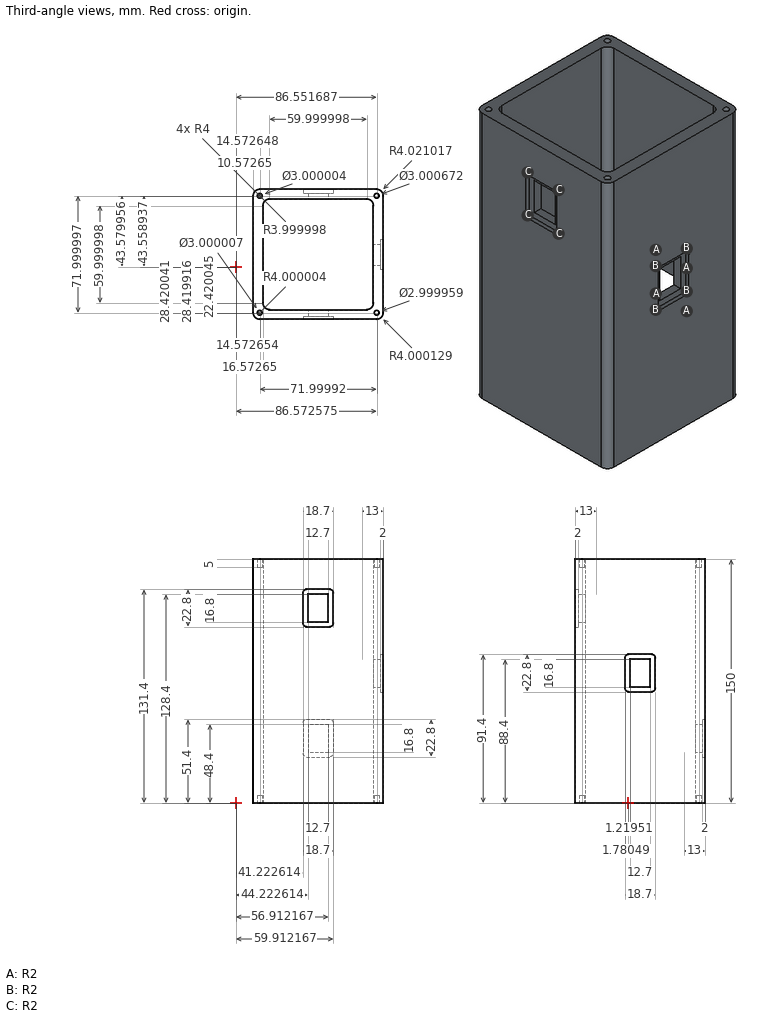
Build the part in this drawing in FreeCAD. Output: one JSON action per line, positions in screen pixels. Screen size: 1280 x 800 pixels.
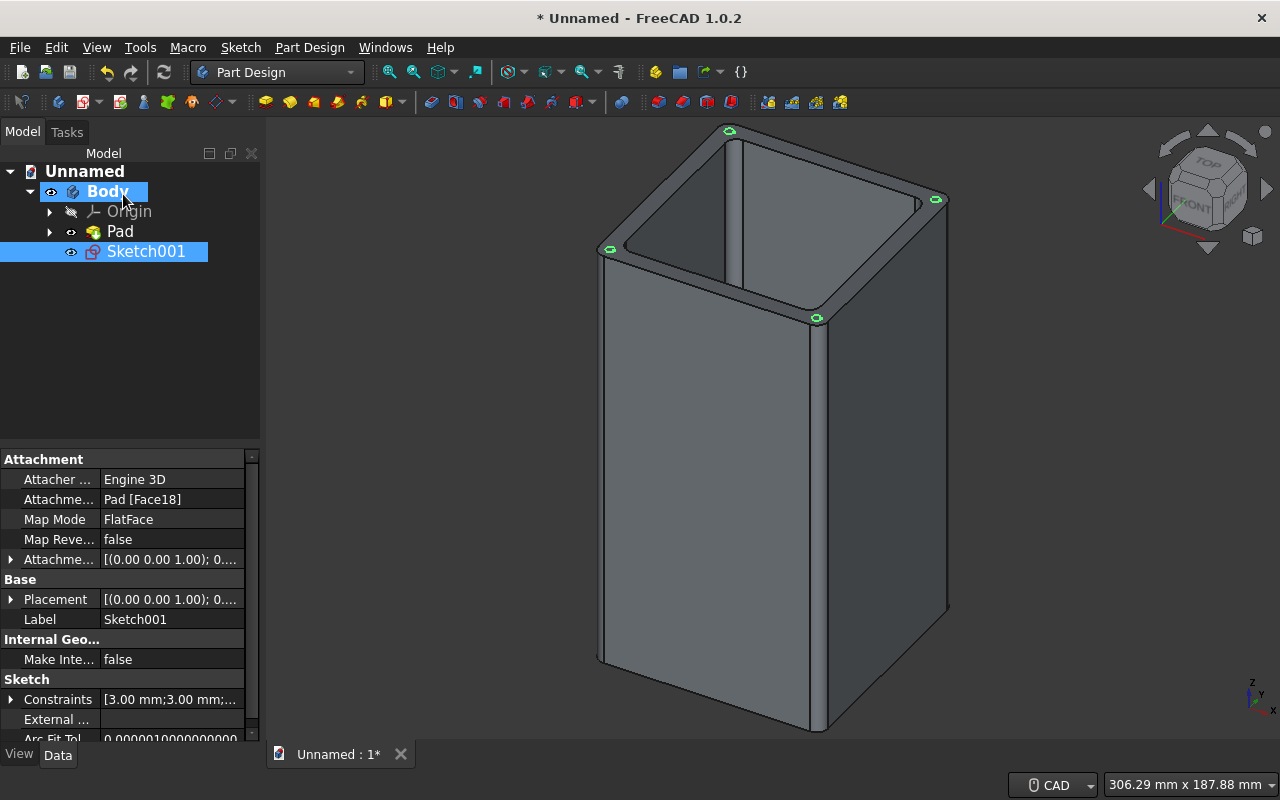
{"action": "left_click", "coordinate": [432, 102]}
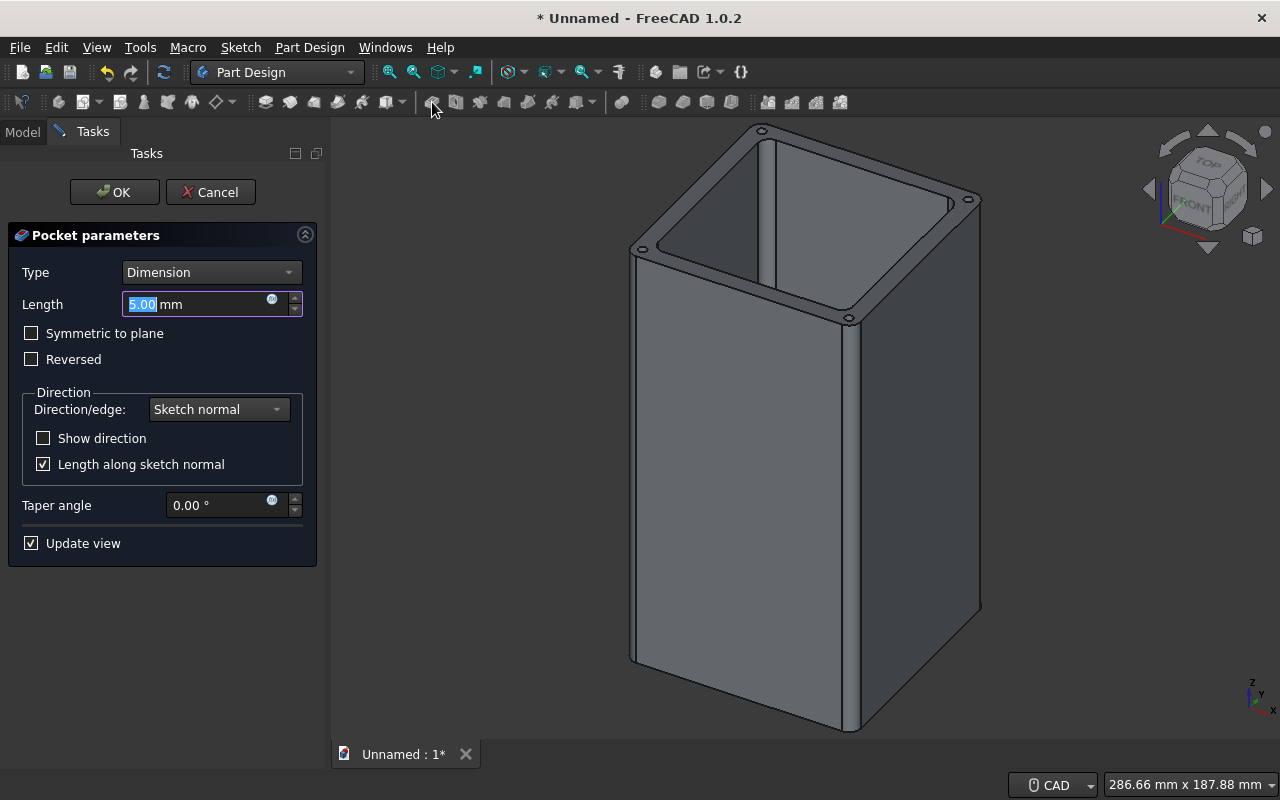
{"action": "type", "text": "5"}
{"action": "key", "text": "Tab"}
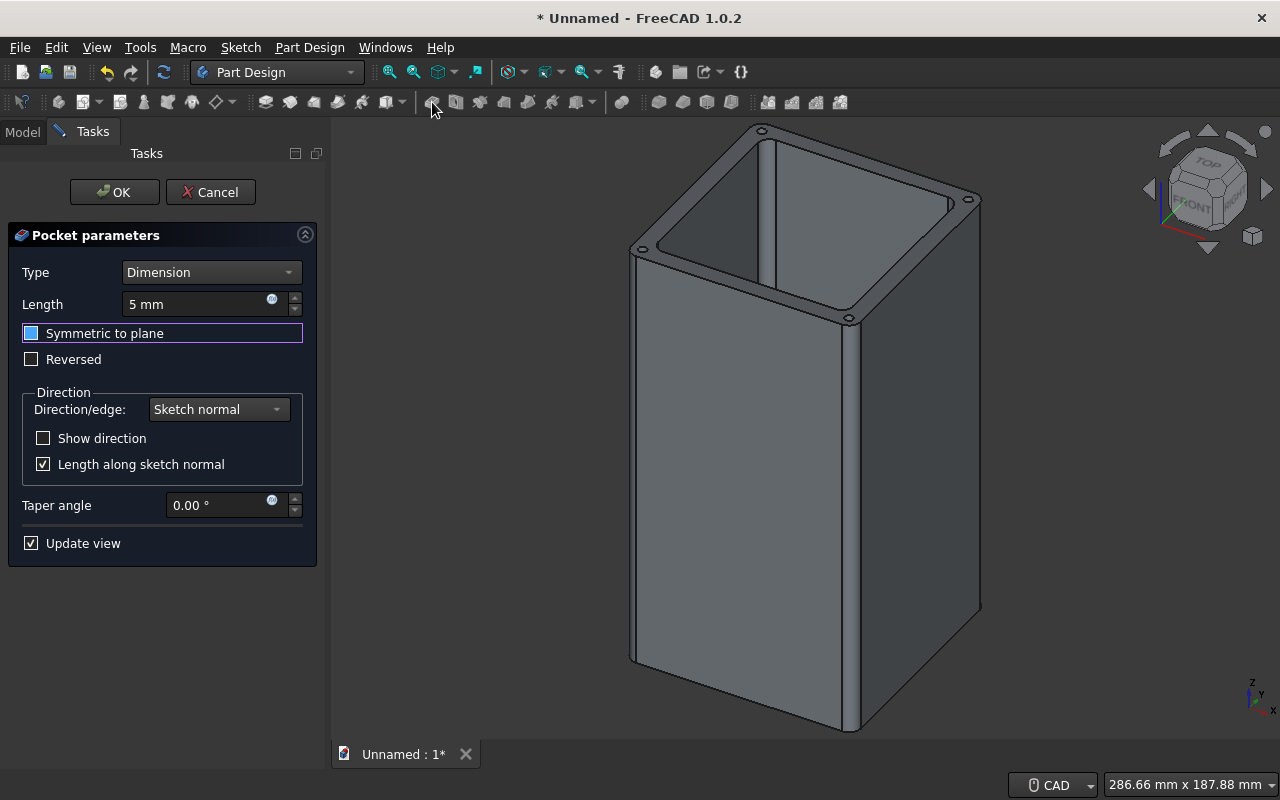
{"action": "left_click", "coordinate": [115, 192]}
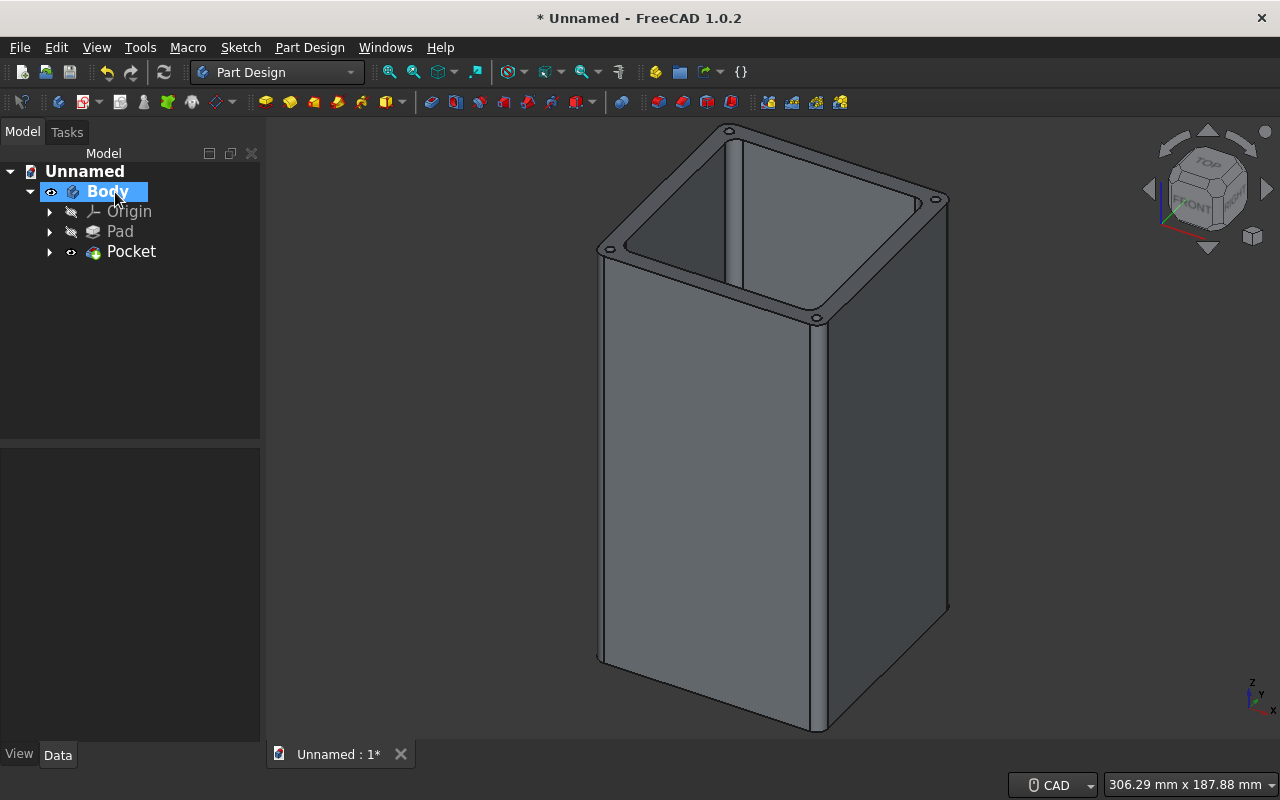
{"action": "left_click", "coordinate": [50, 212]}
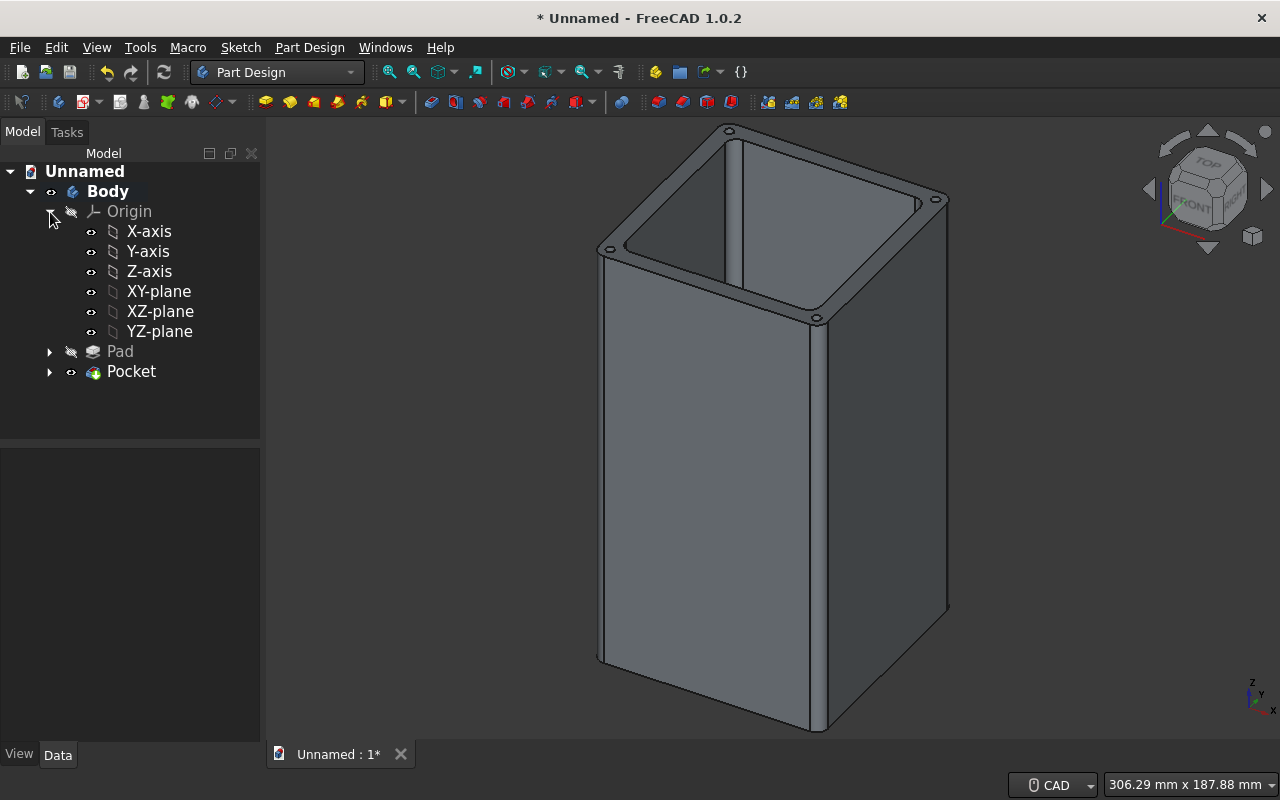
{"action": "left_click", "coordinate": [136, 292]}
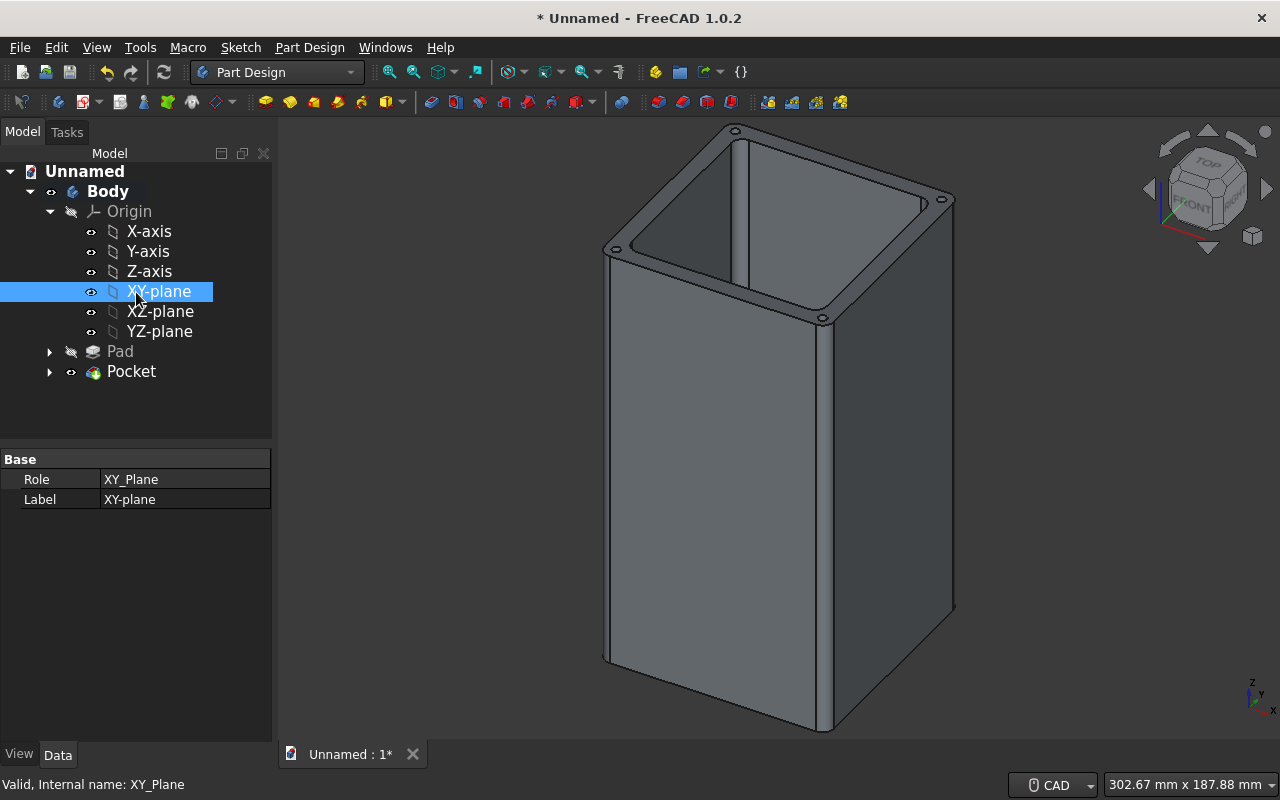
{"action": "left_click", "coordinate": [216, 102]}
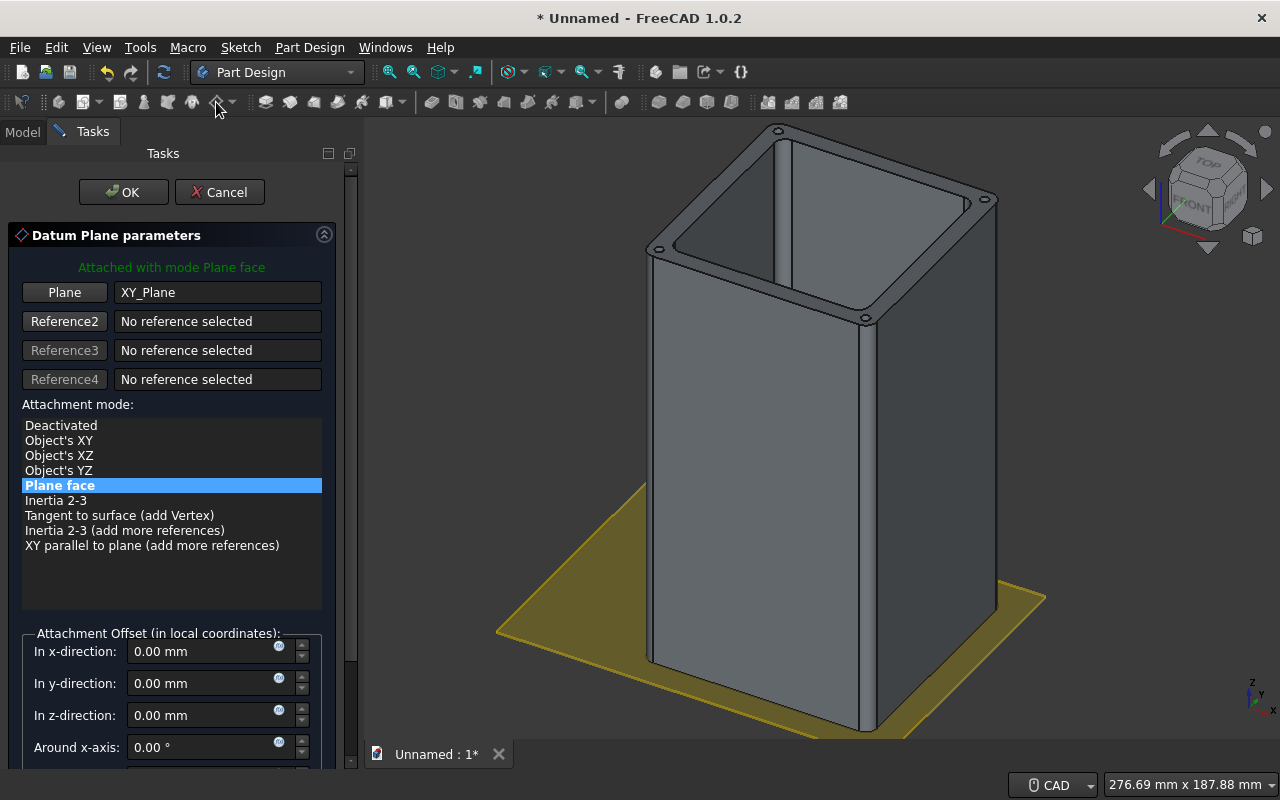
{"action": "triple_click", "coordinate": [210, 715]}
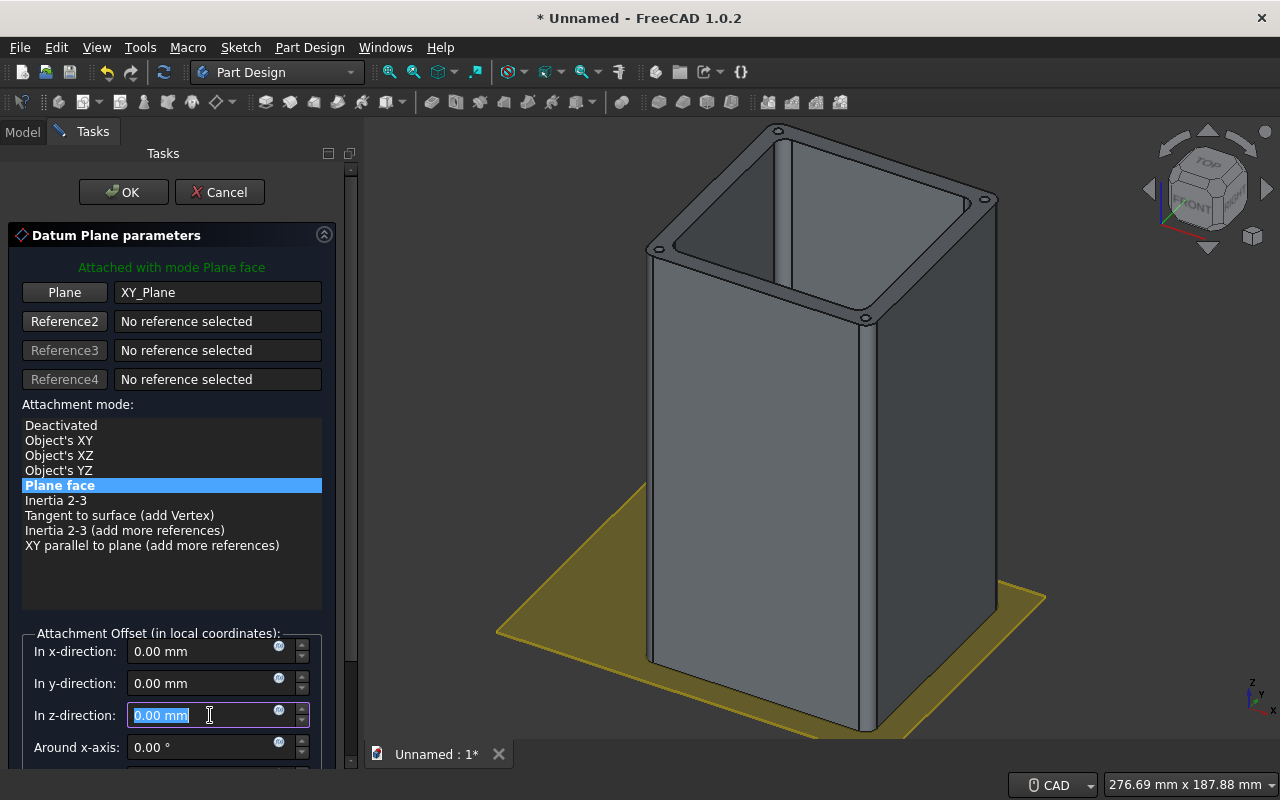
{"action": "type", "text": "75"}
{"action": "key", "text": "Tab"}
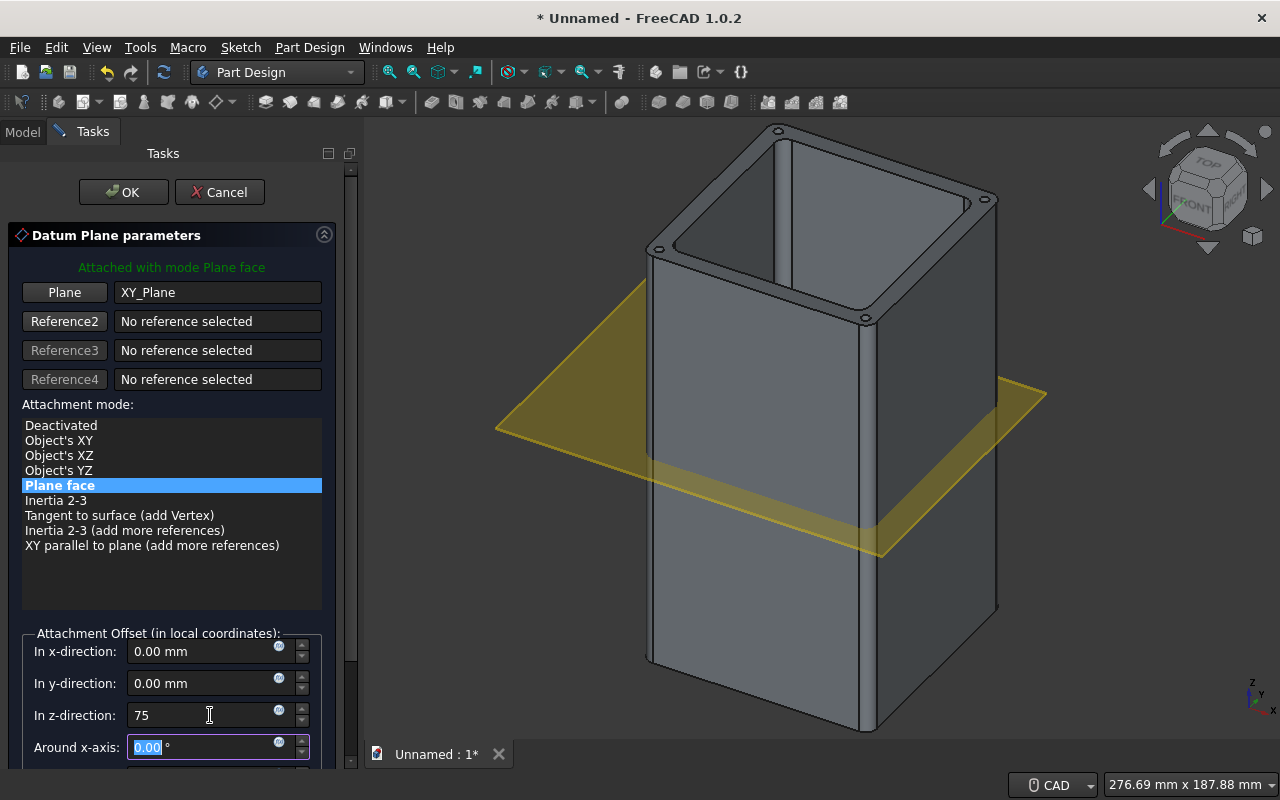
{"action": "left_click", "coordinate": [124, 192]}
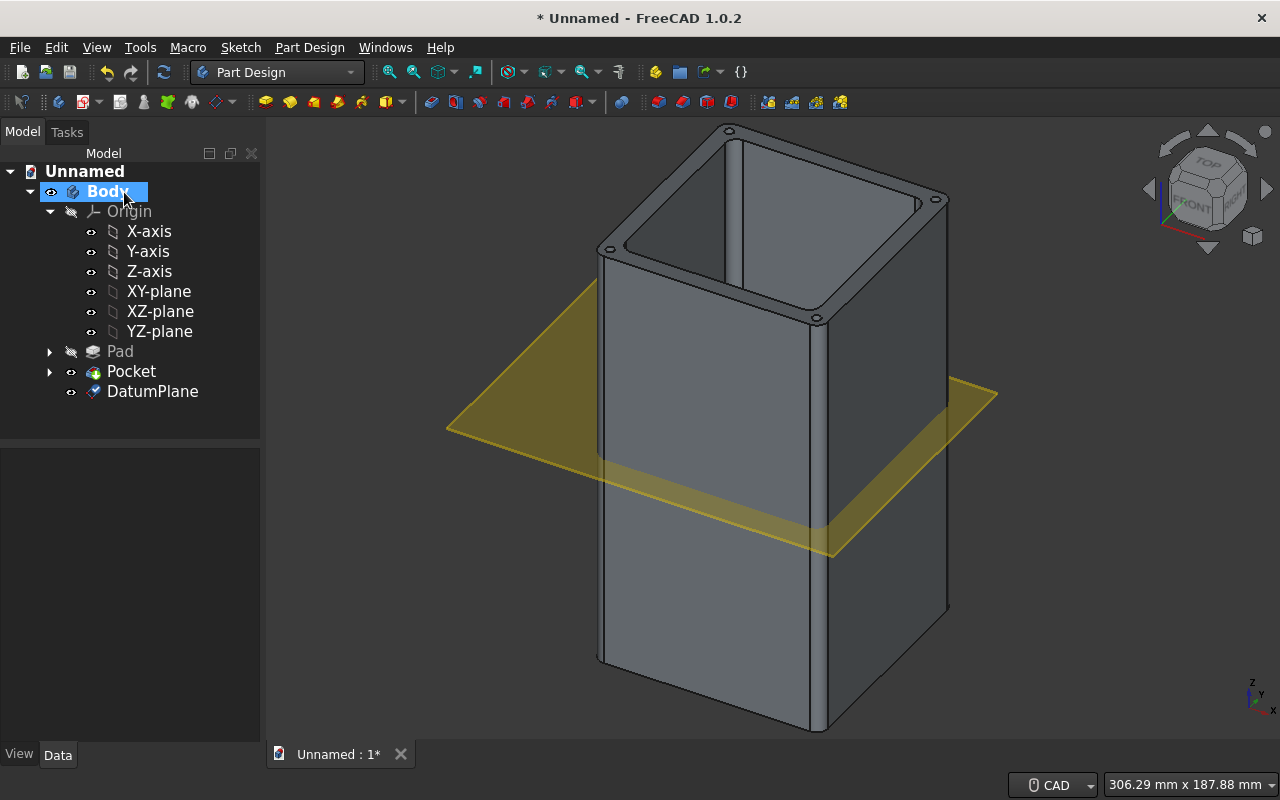
{"action": "left_click", "coordinate": [116, 372]}